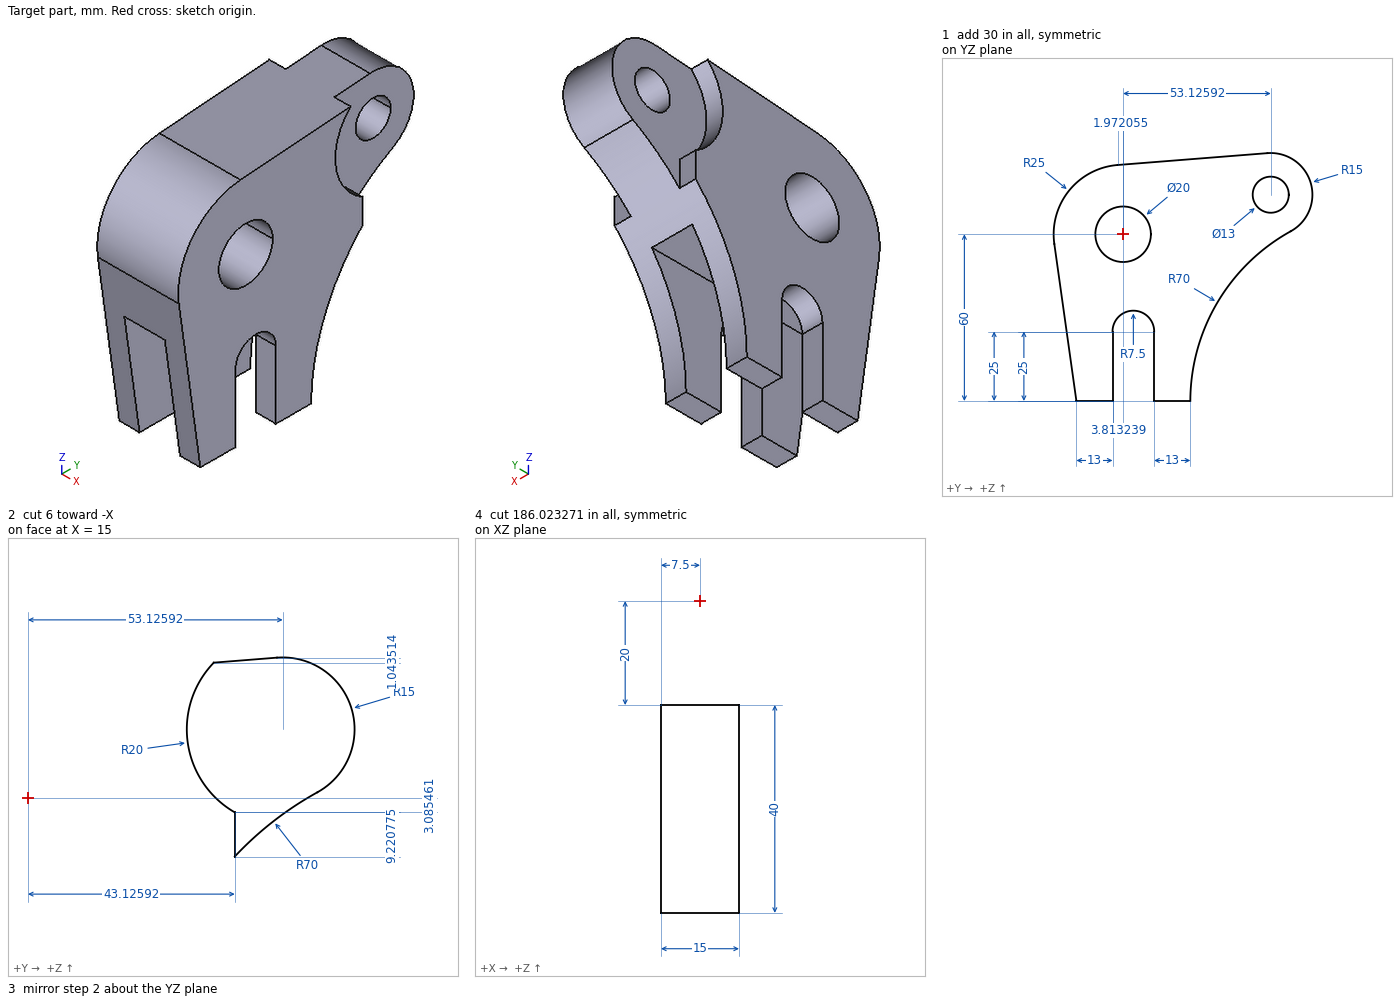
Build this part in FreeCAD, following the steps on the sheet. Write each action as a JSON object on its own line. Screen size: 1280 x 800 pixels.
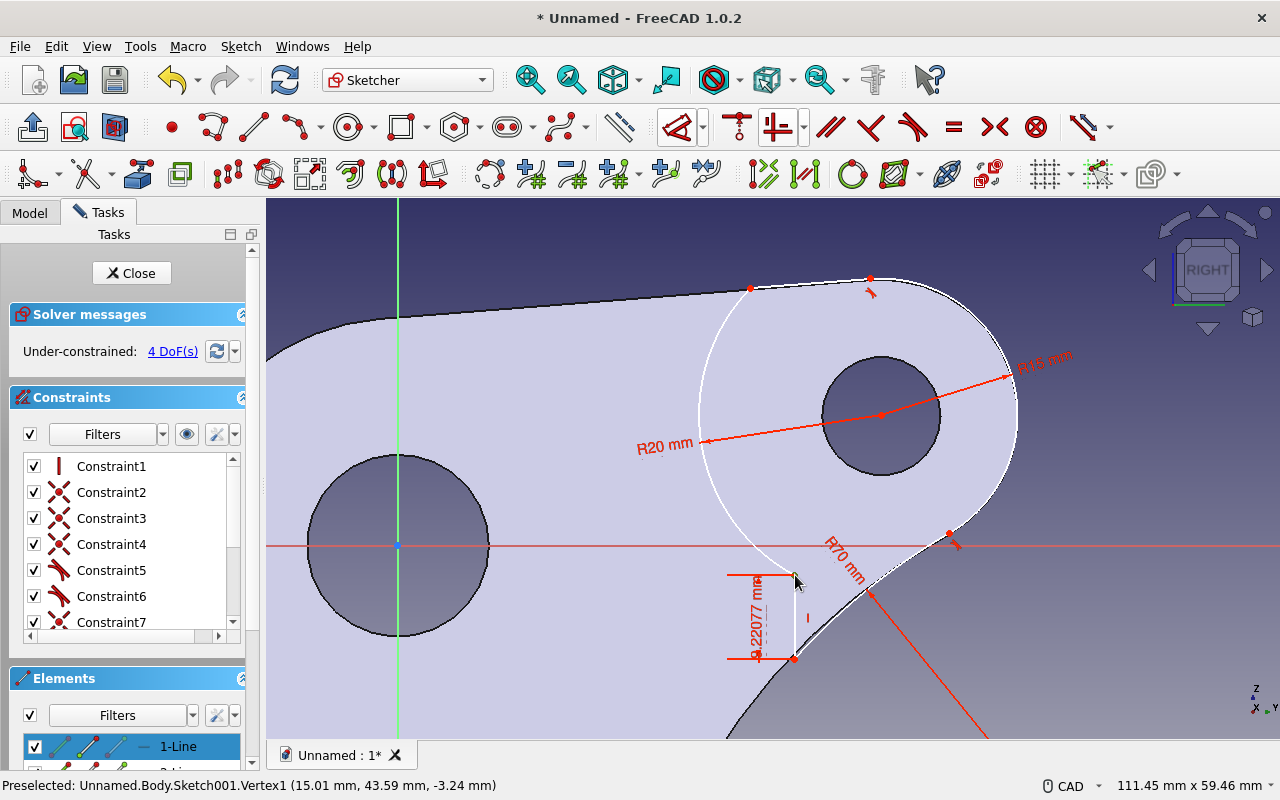
{"action": "left_click", "coordinate": [702, 128]}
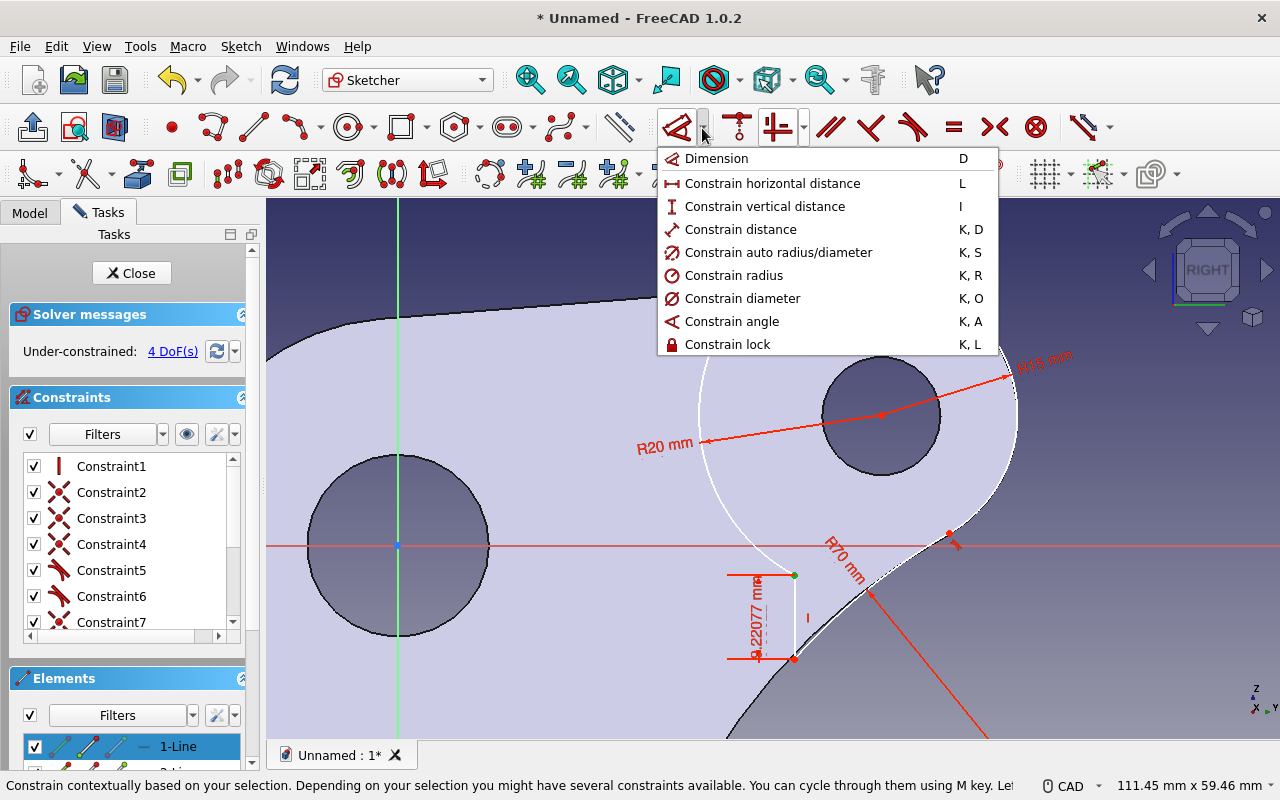
{"action": "left_click", "coordinate": [828, 184]}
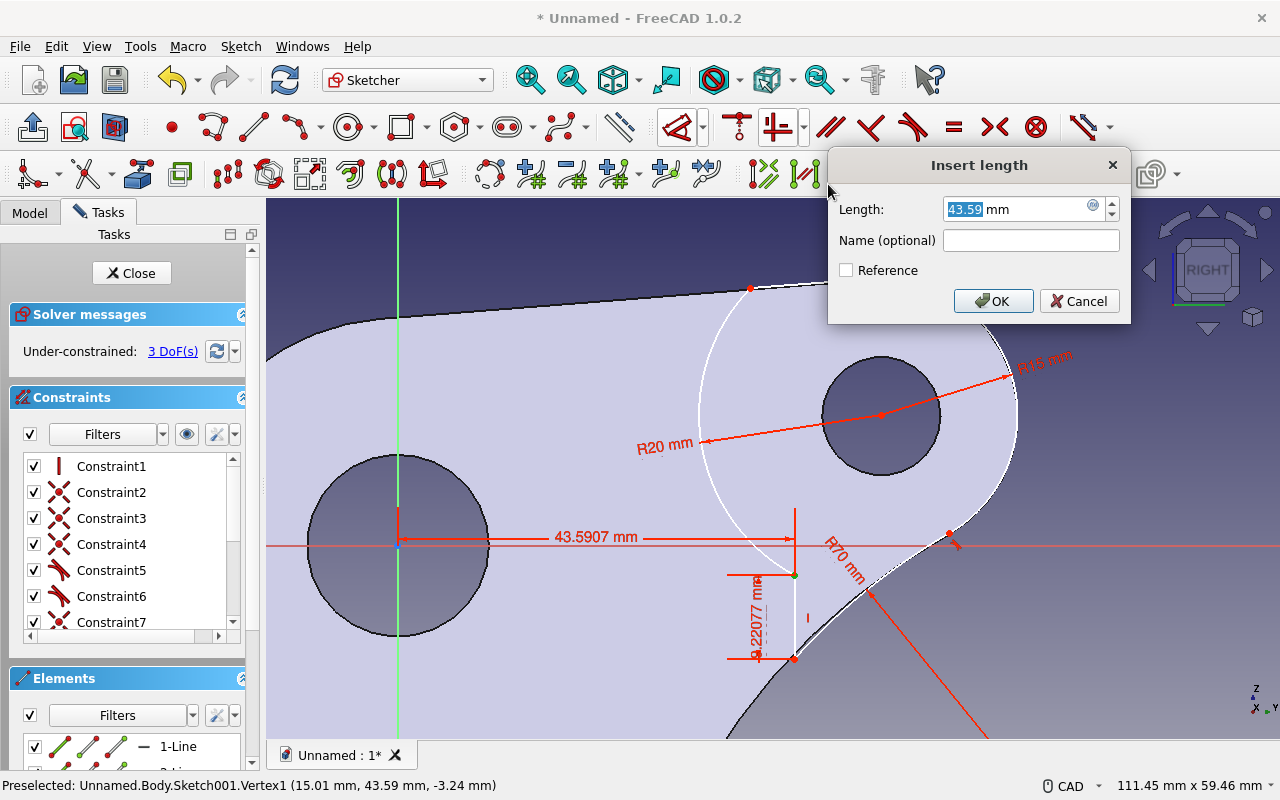
{"action": "type", "text": "43.12592"}
{"action": "key", "text": "Return"}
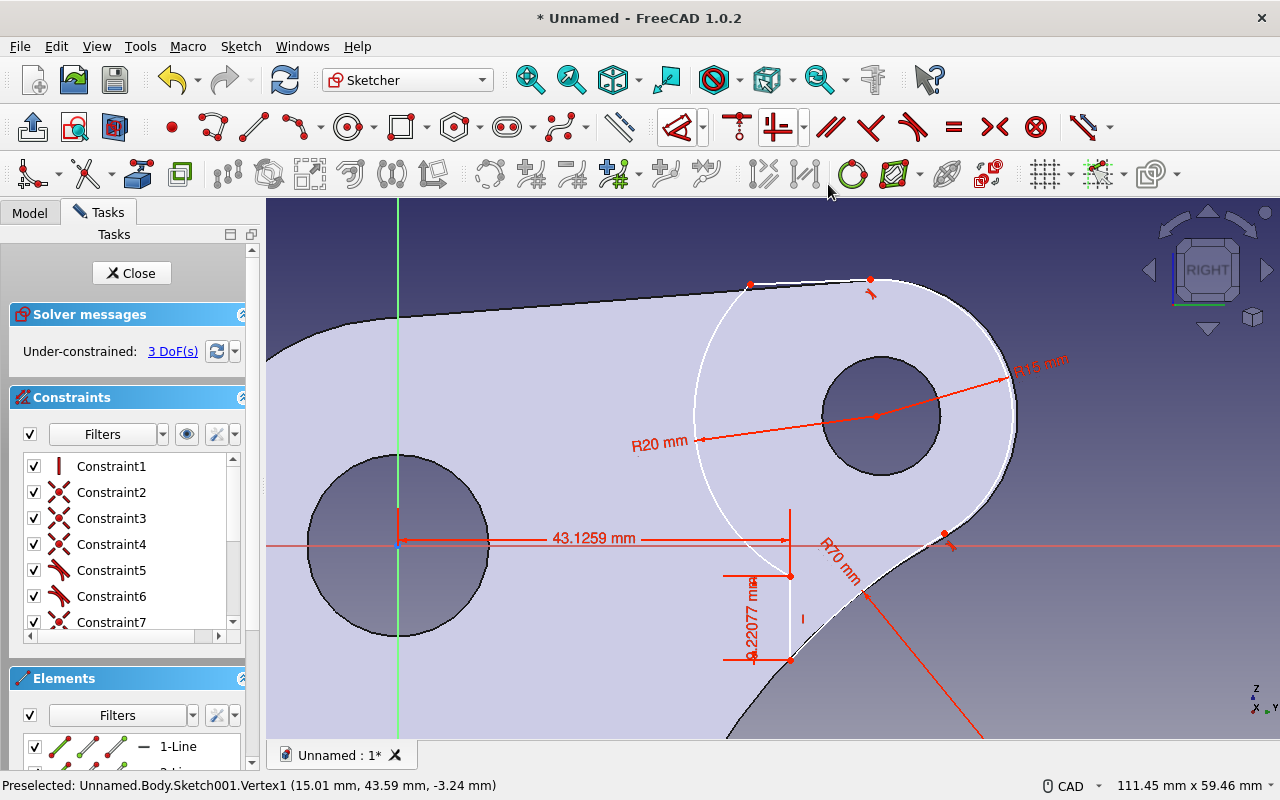
{"action": "scroll", "coordinate": [790, 576], "scroll_direction": "up", "scroll_amount": 2}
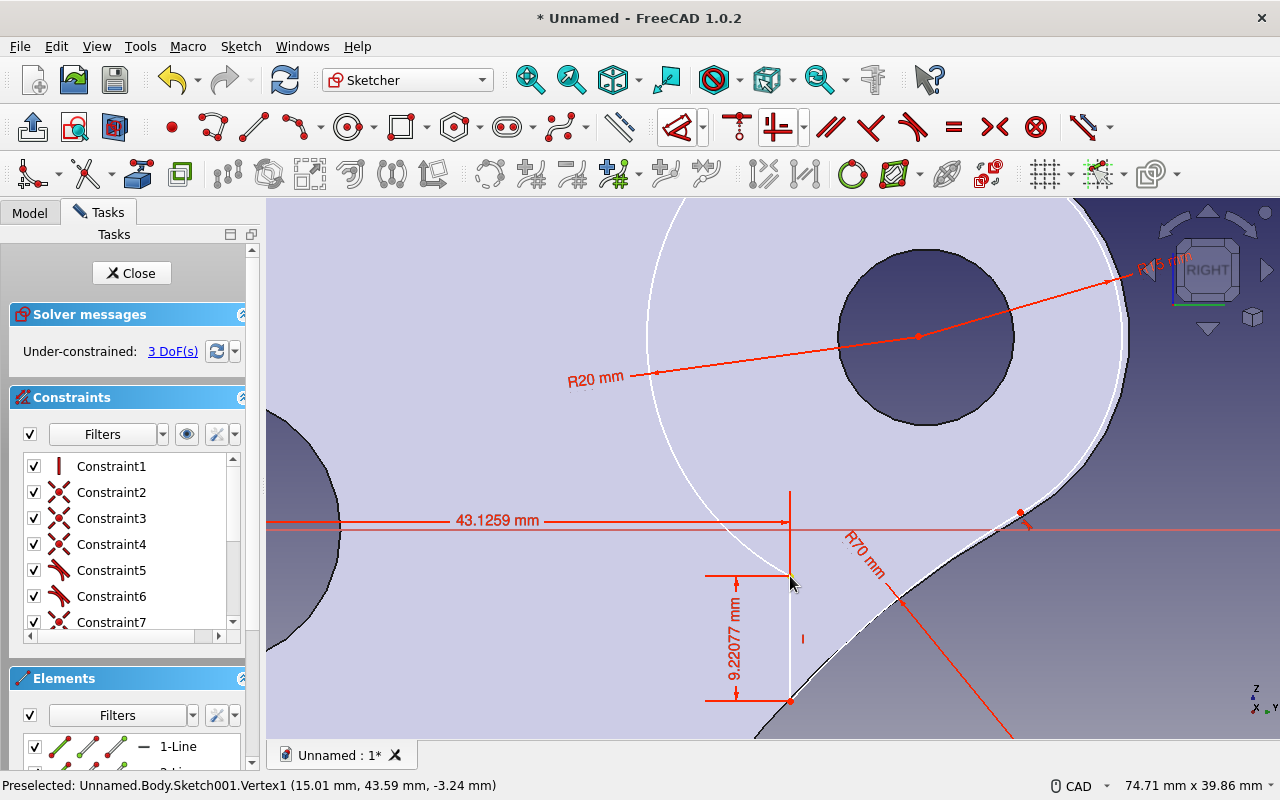
{"action": "left_click", "coordinate": [790, 576]}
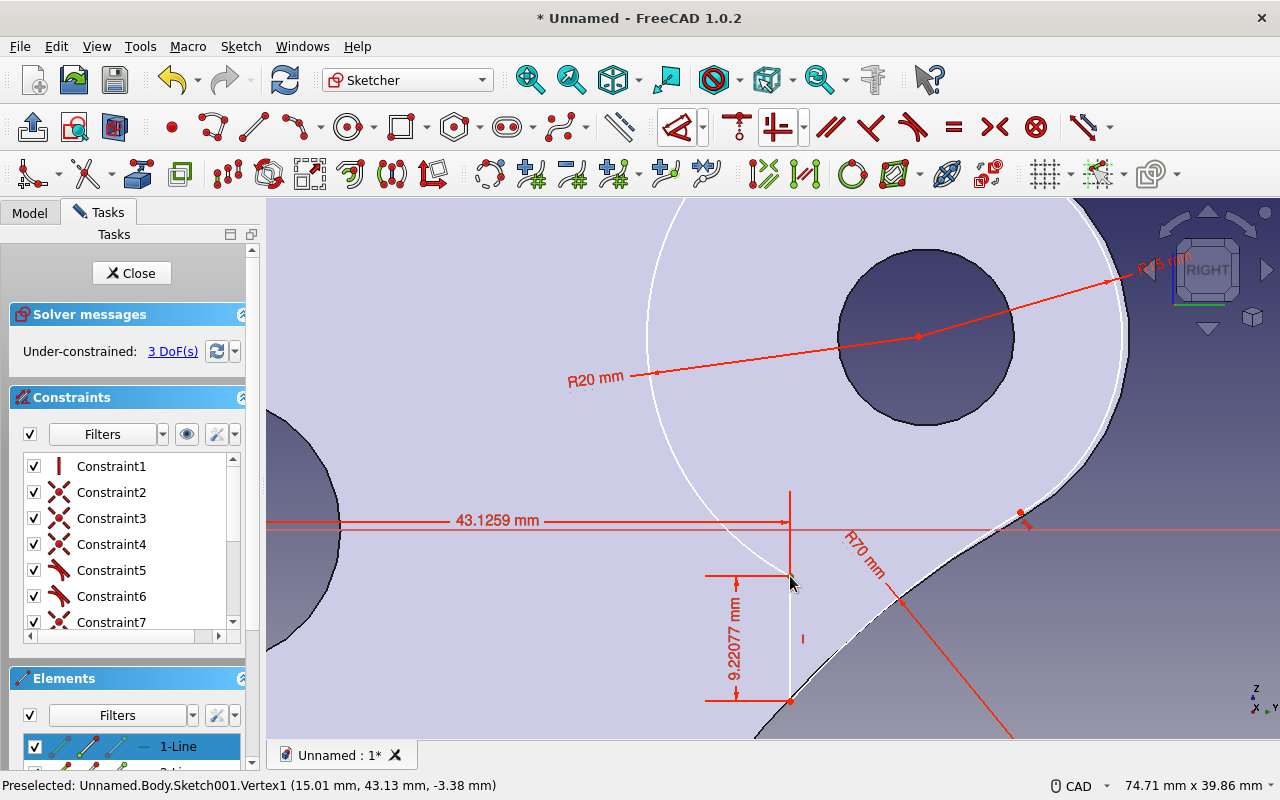
{"action": "left_click", "coordinate": [702, 128]}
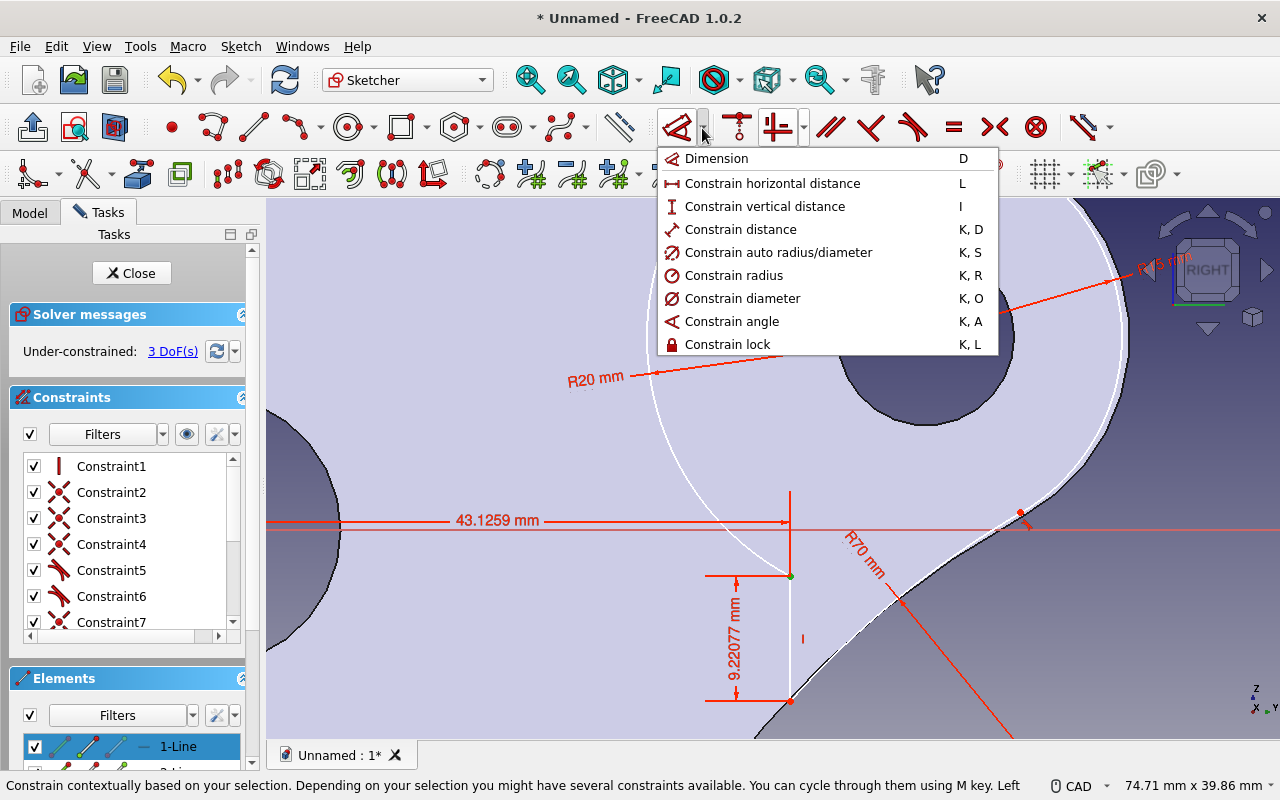
{"action": "left_click", "coordinate": [828, 206]}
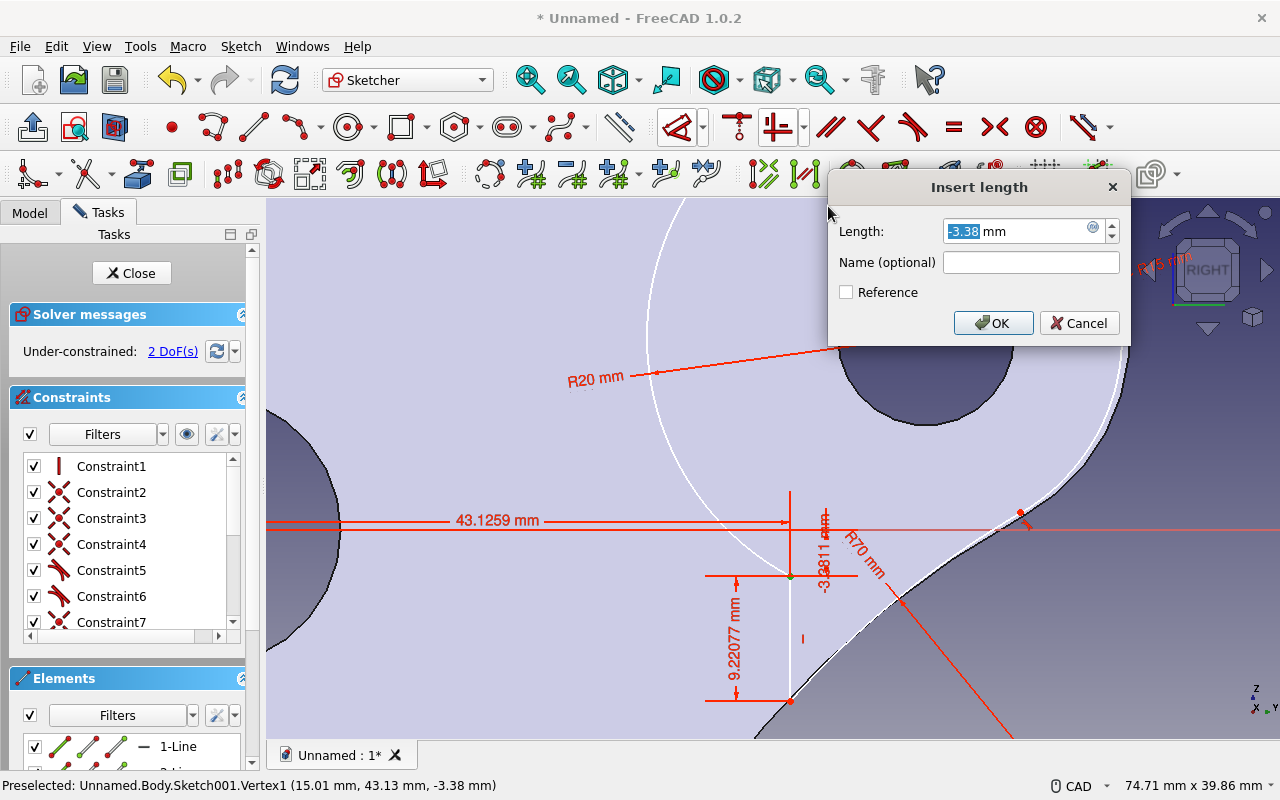
{"action": "type", "text": "-3.085461"}
{"action": "key", "text": "Return"}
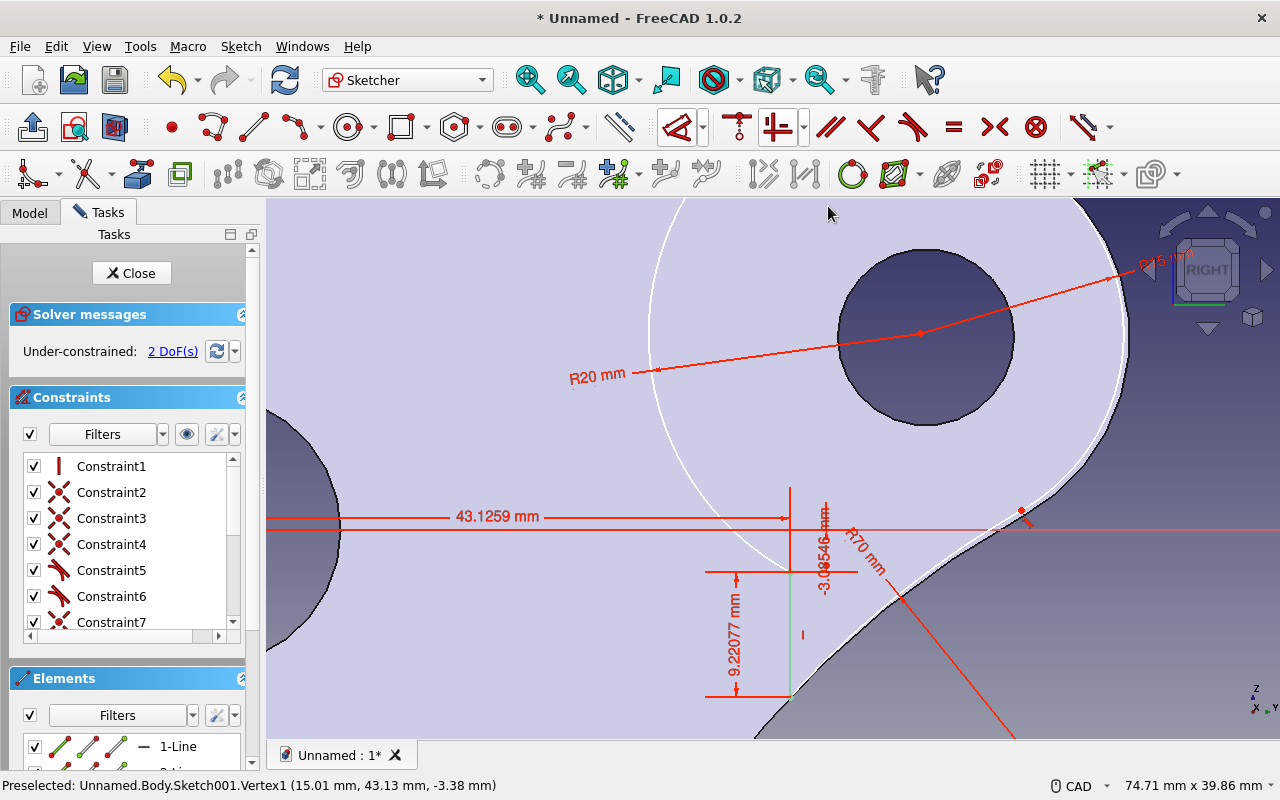
{"action": "scroll", "coordinate": [789, 576], "scroll_direction": "down", "scroll_amount": 2}